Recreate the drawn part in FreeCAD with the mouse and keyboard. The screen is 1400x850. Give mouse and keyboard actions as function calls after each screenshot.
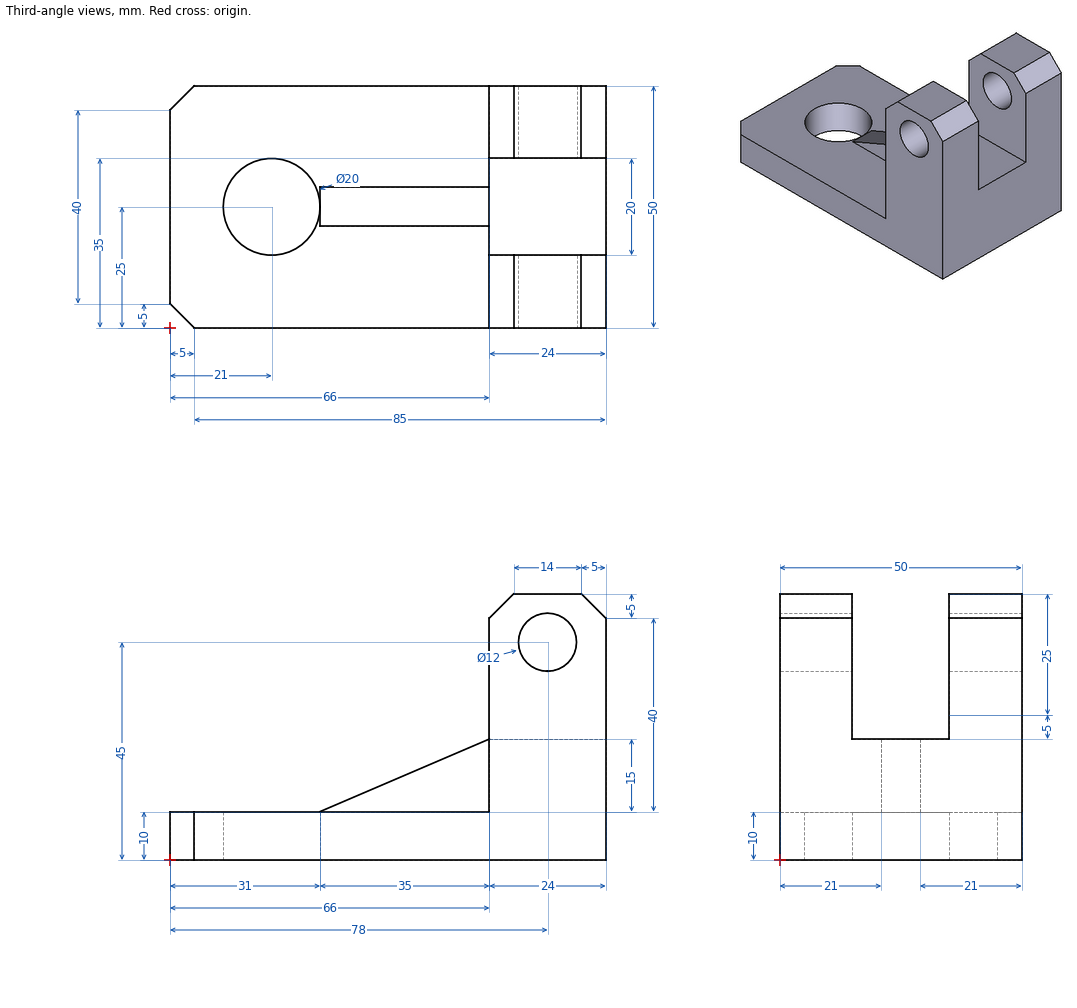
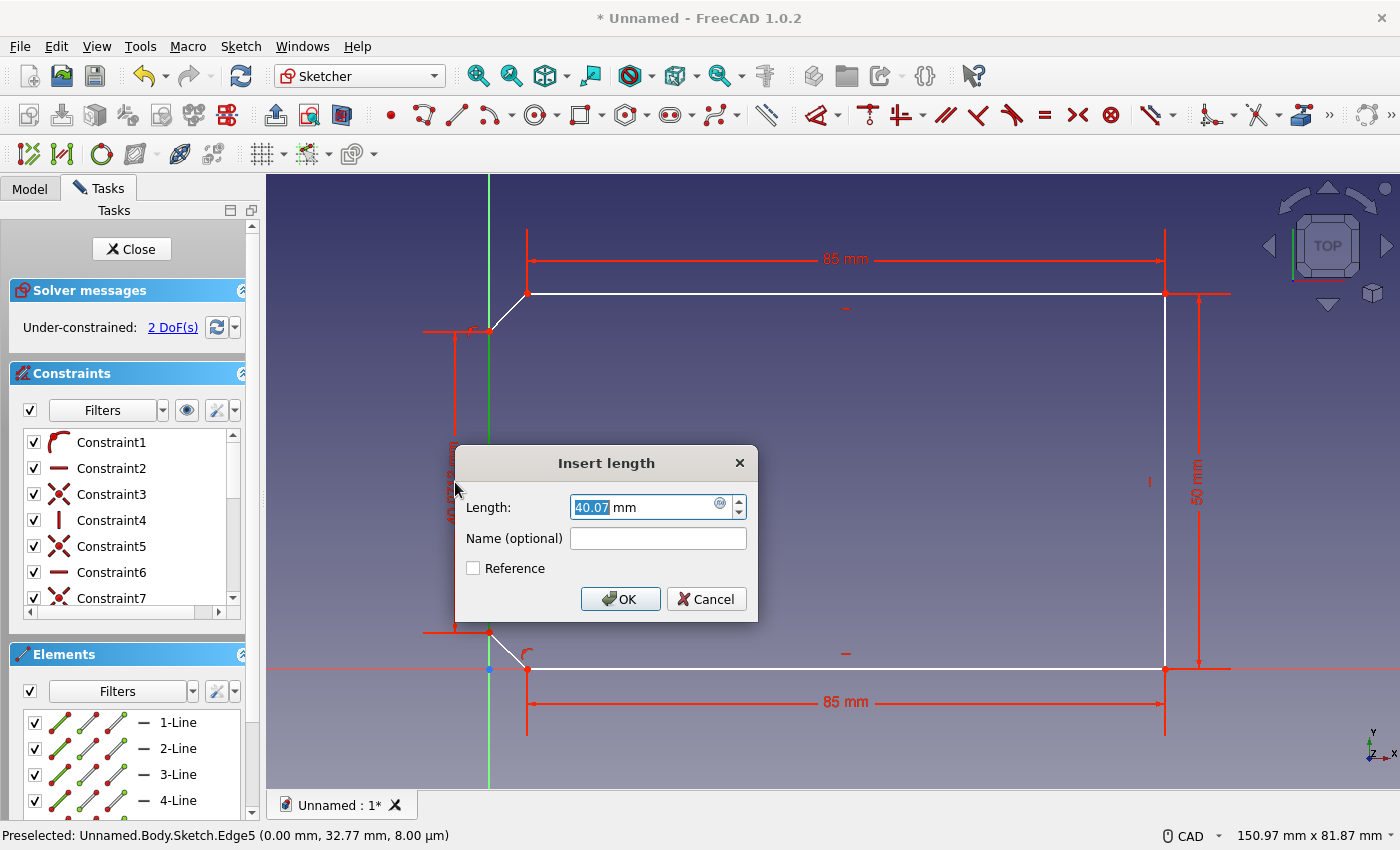
text(40)
key(Return)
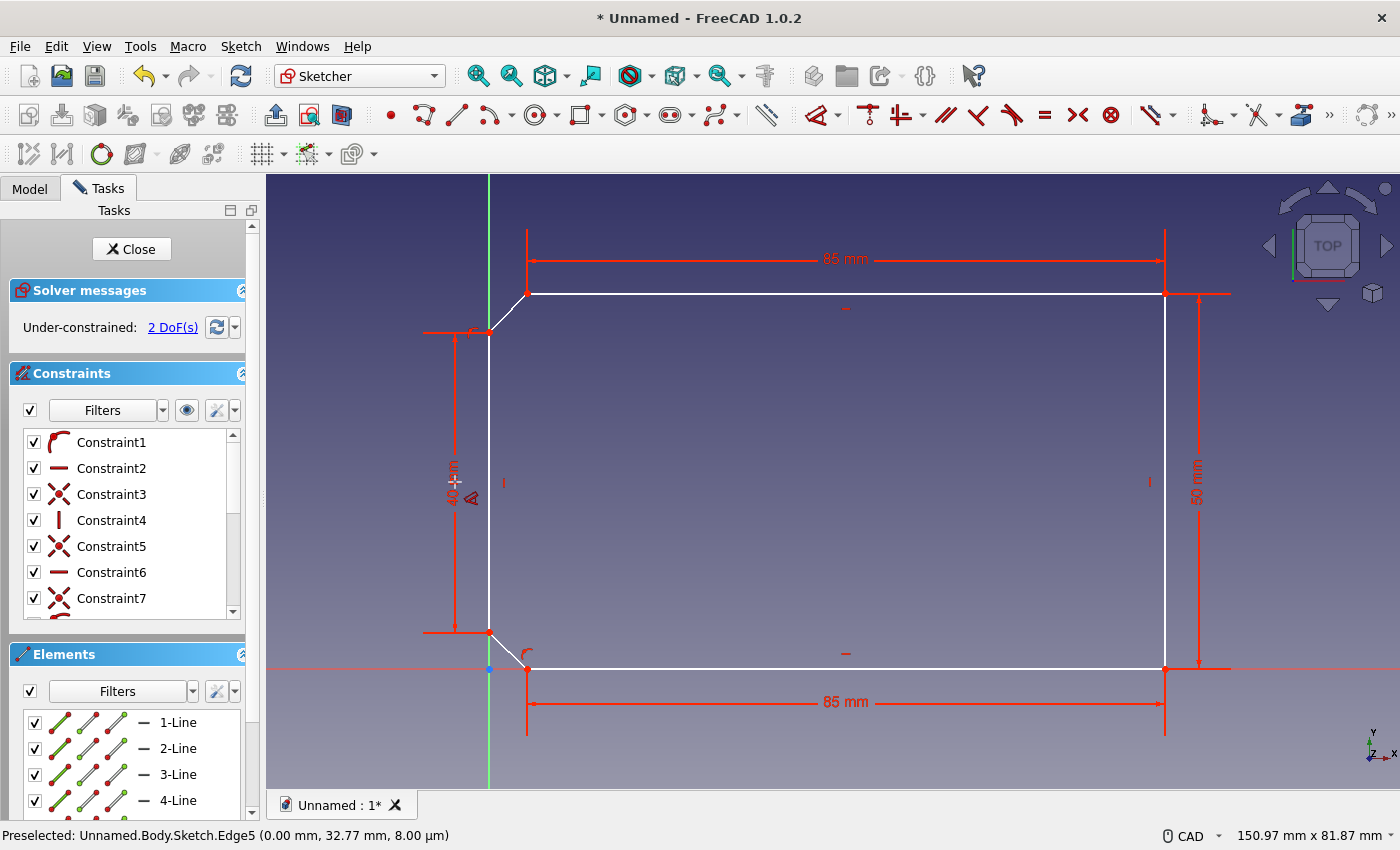
click(527, 669)
click(508, 703)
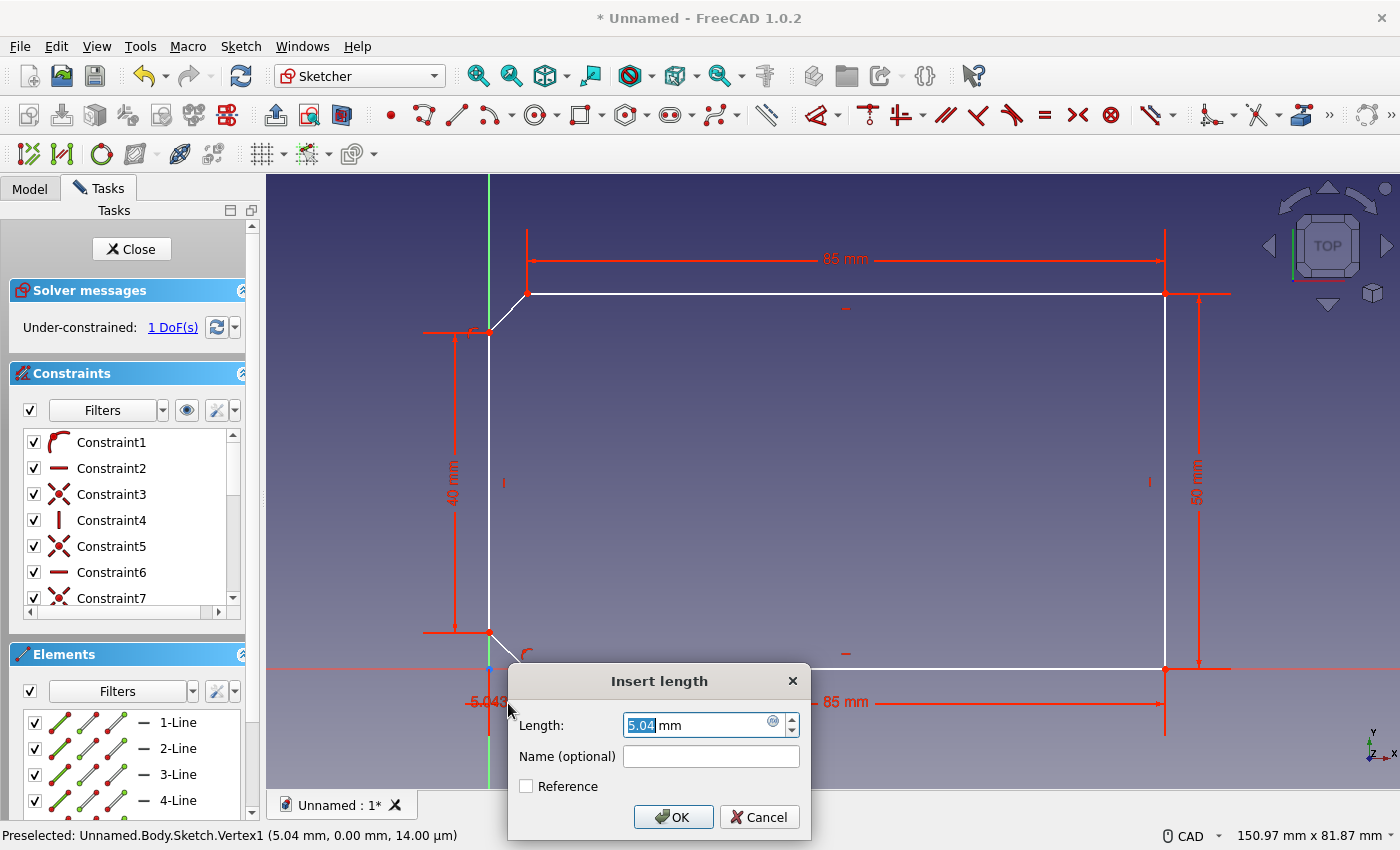
text(5)
key(Return)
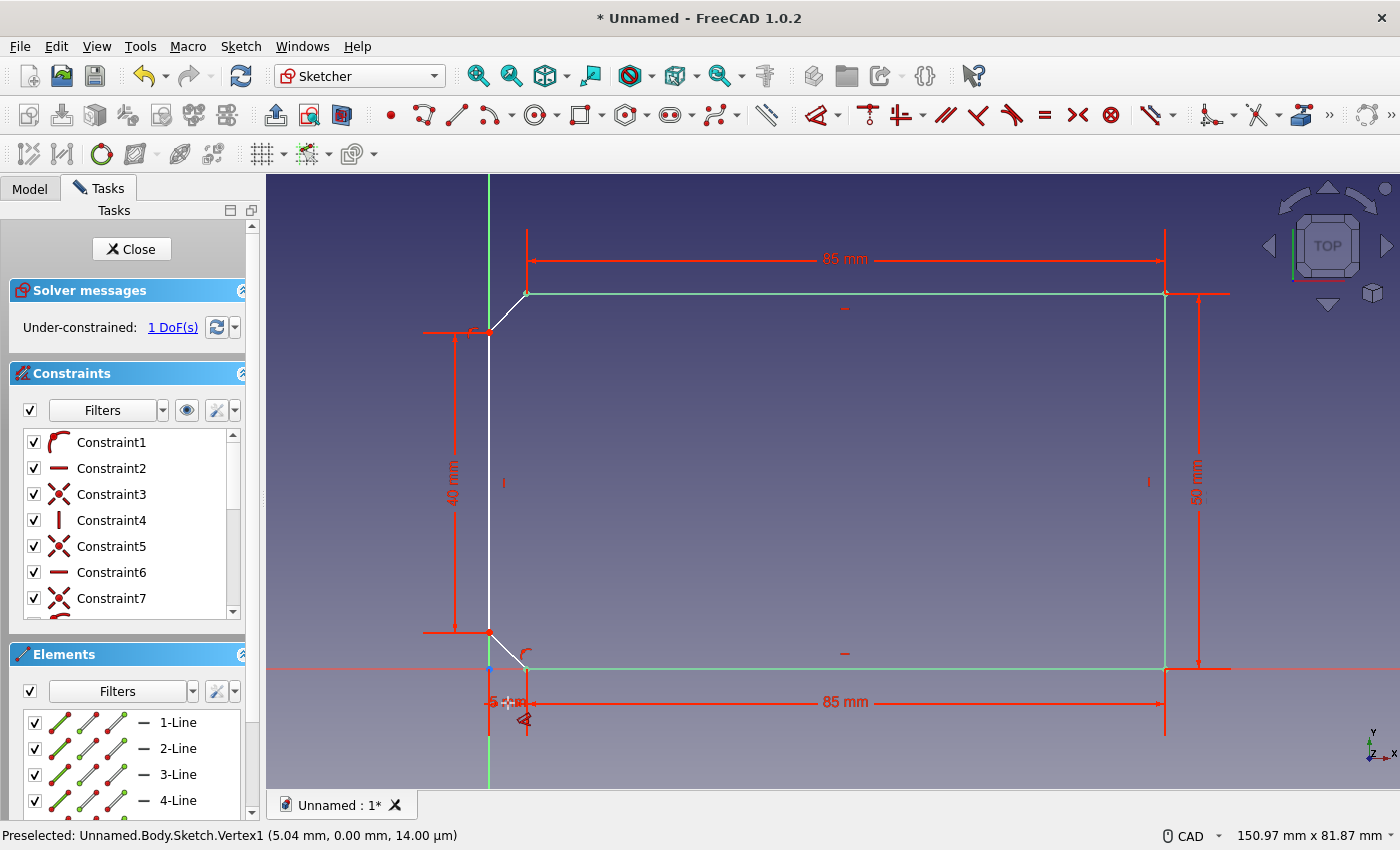
click(489, 633)
click(455, 651)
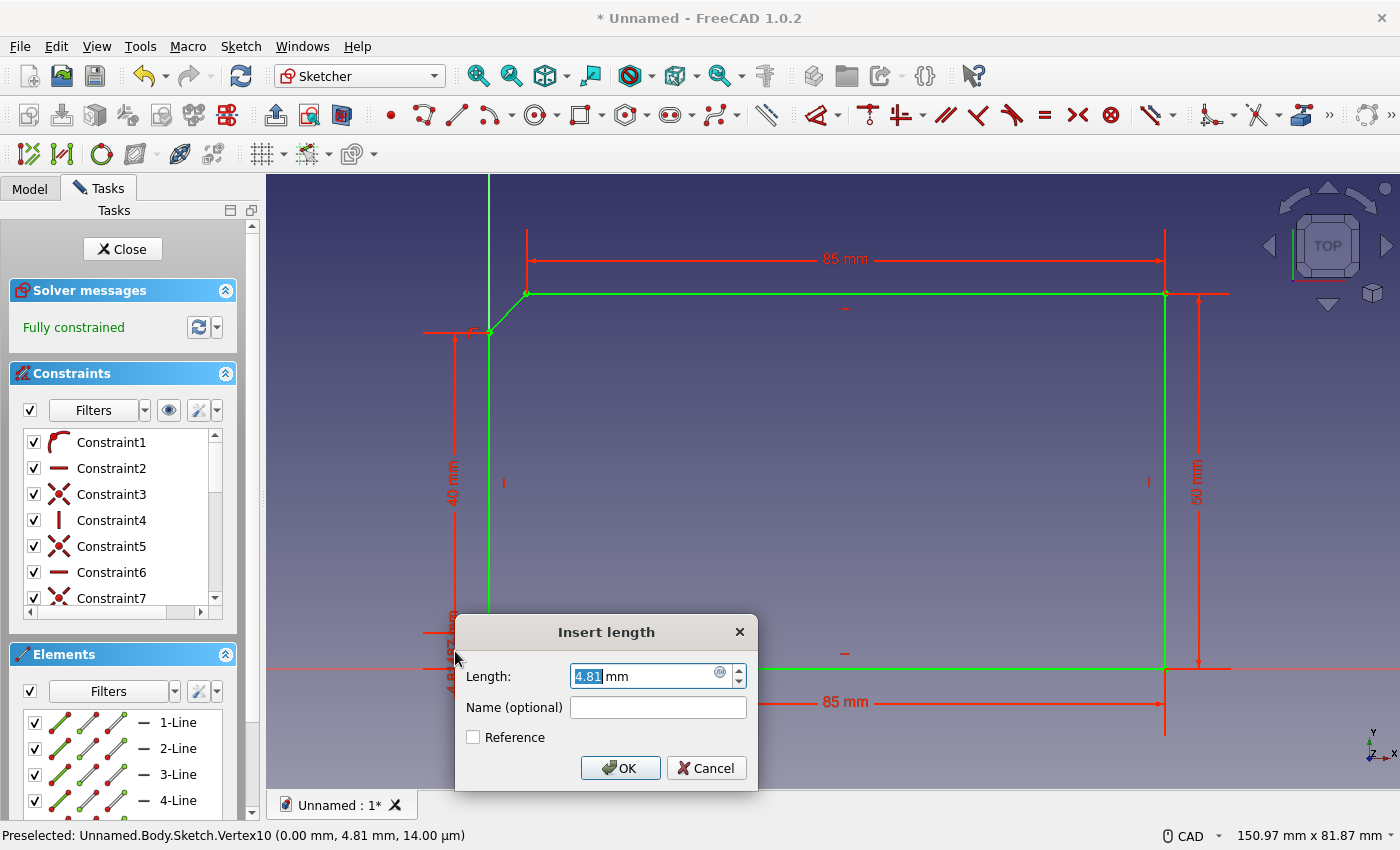
text(5)
key(Return)
key(Escape)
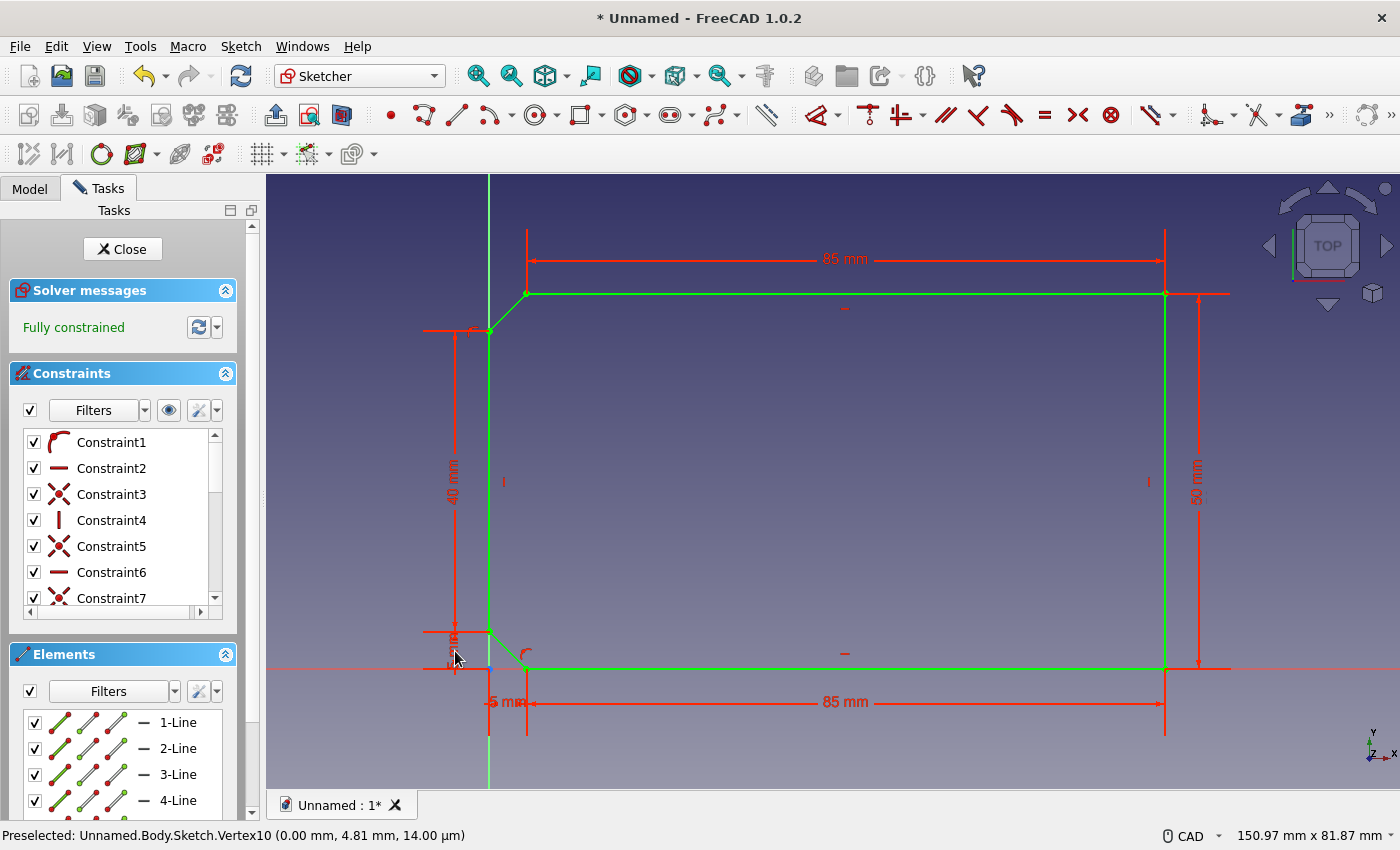
click(123, 249)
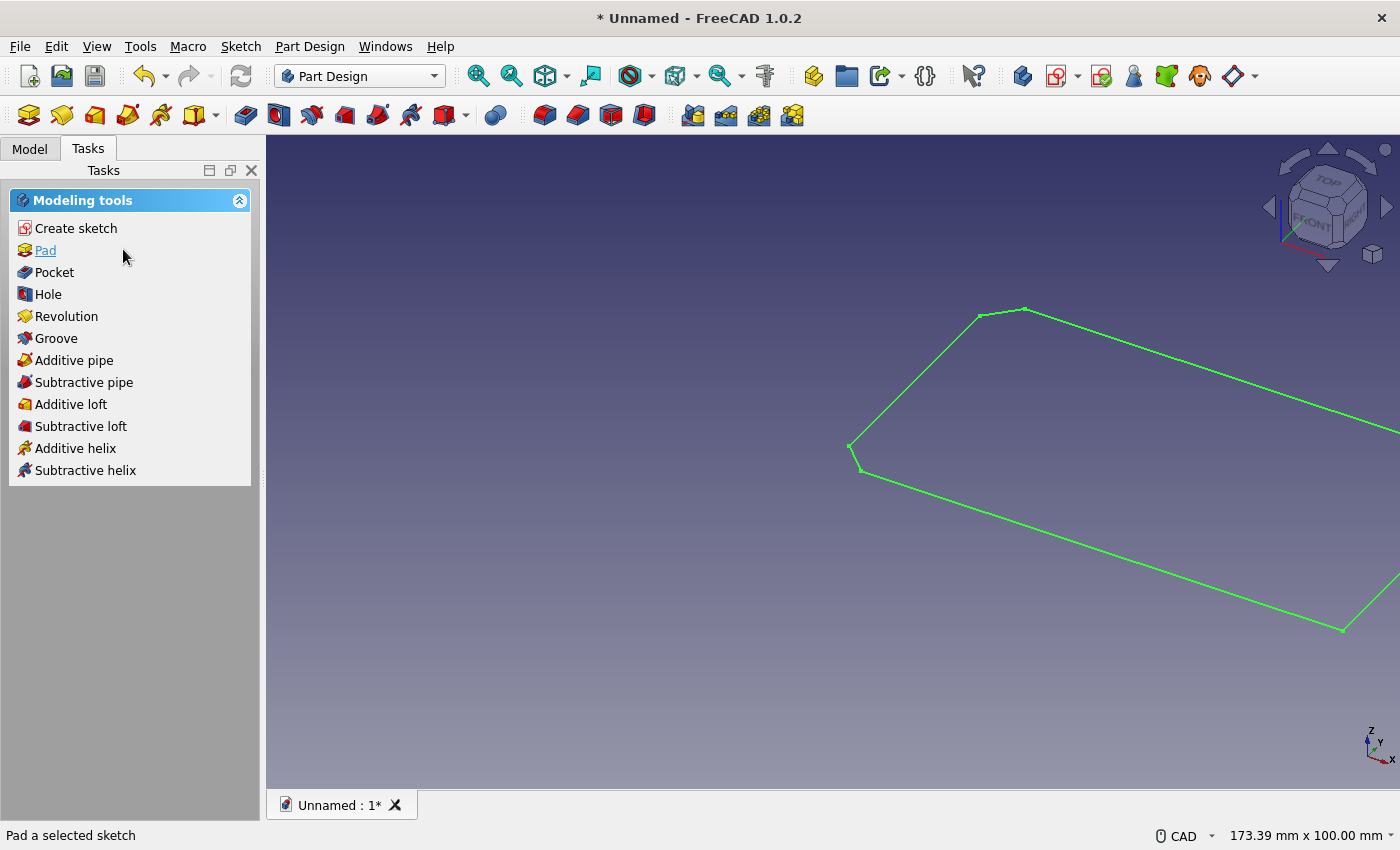
click(29, 116)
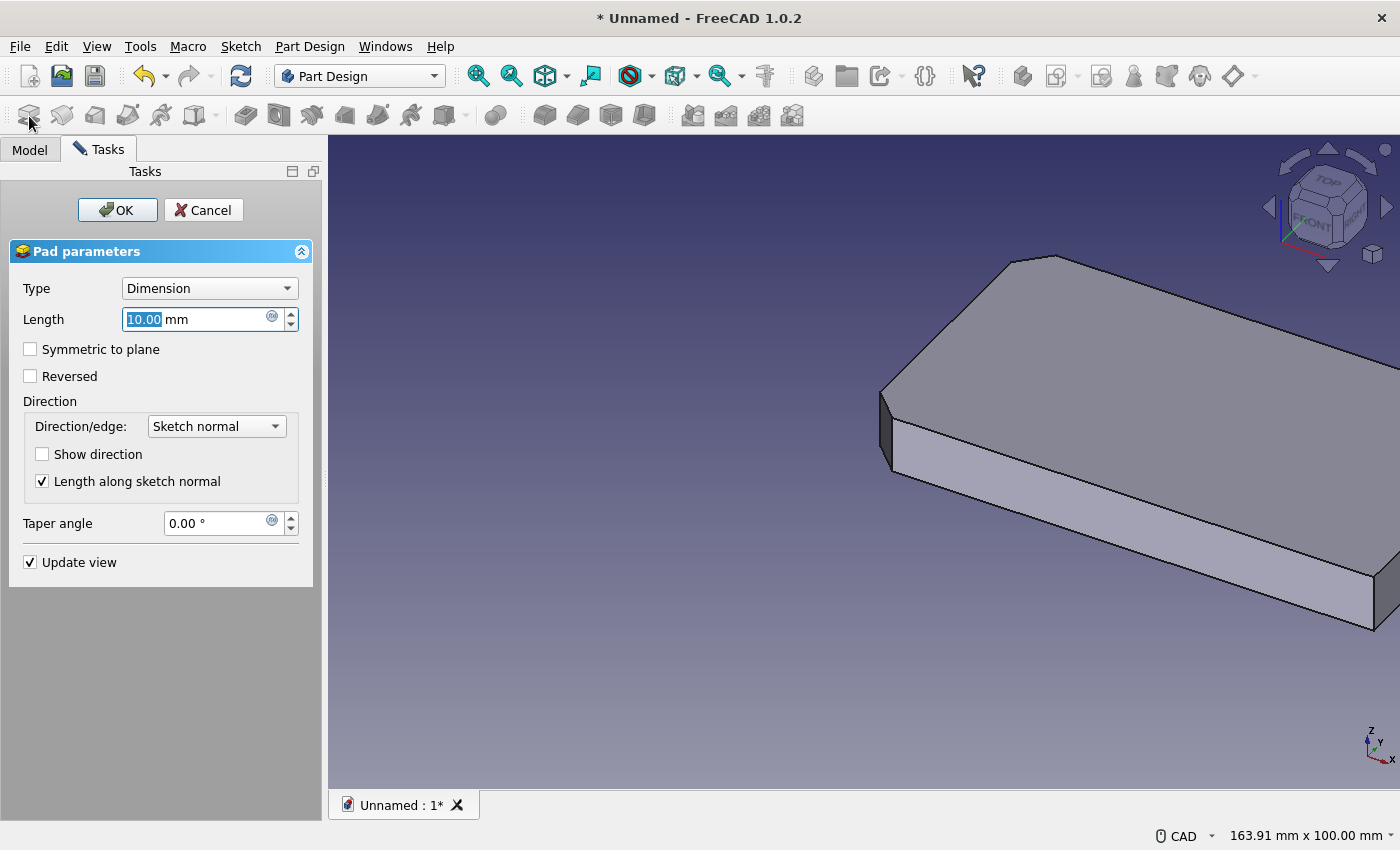
text(10)
key(Tab)